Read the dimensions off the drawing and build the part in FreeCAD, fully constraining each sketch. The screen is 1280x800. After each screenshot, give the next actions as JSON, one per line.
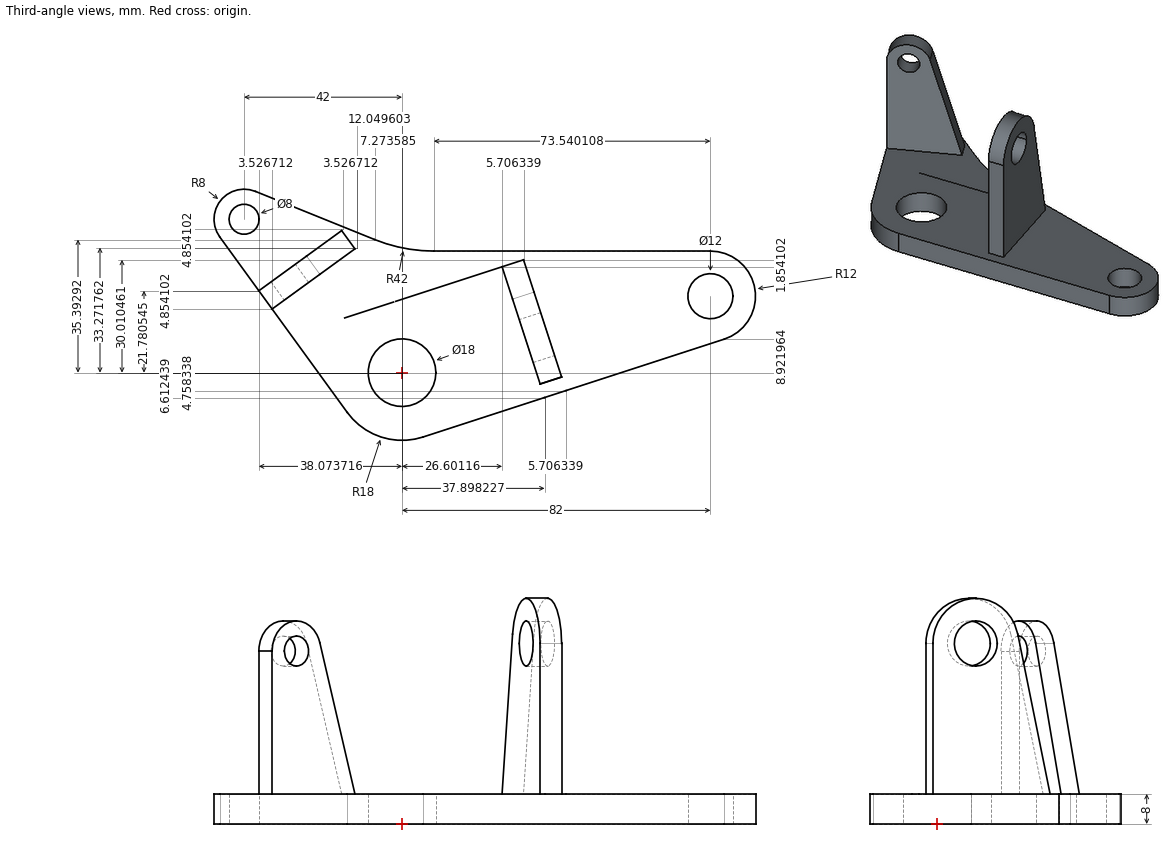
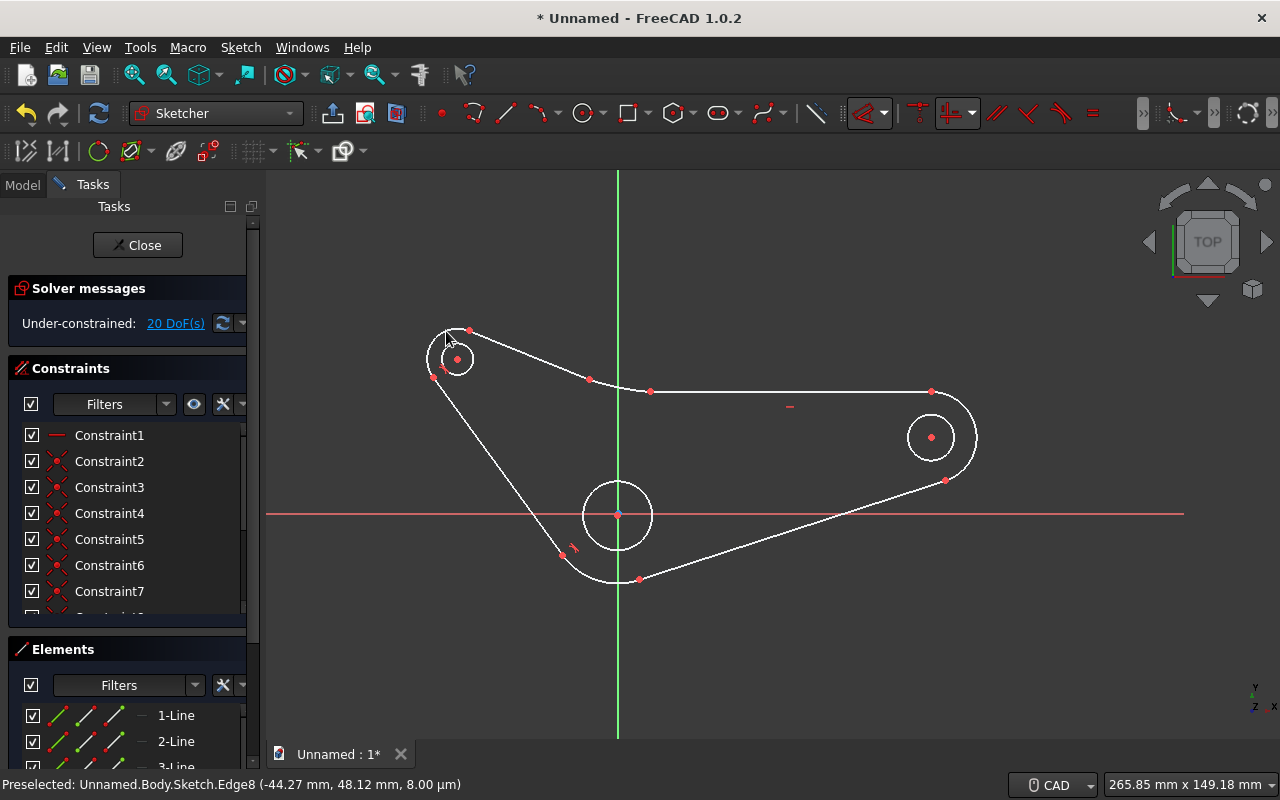
{"action": "left_click", "coordinate": [731, 550]}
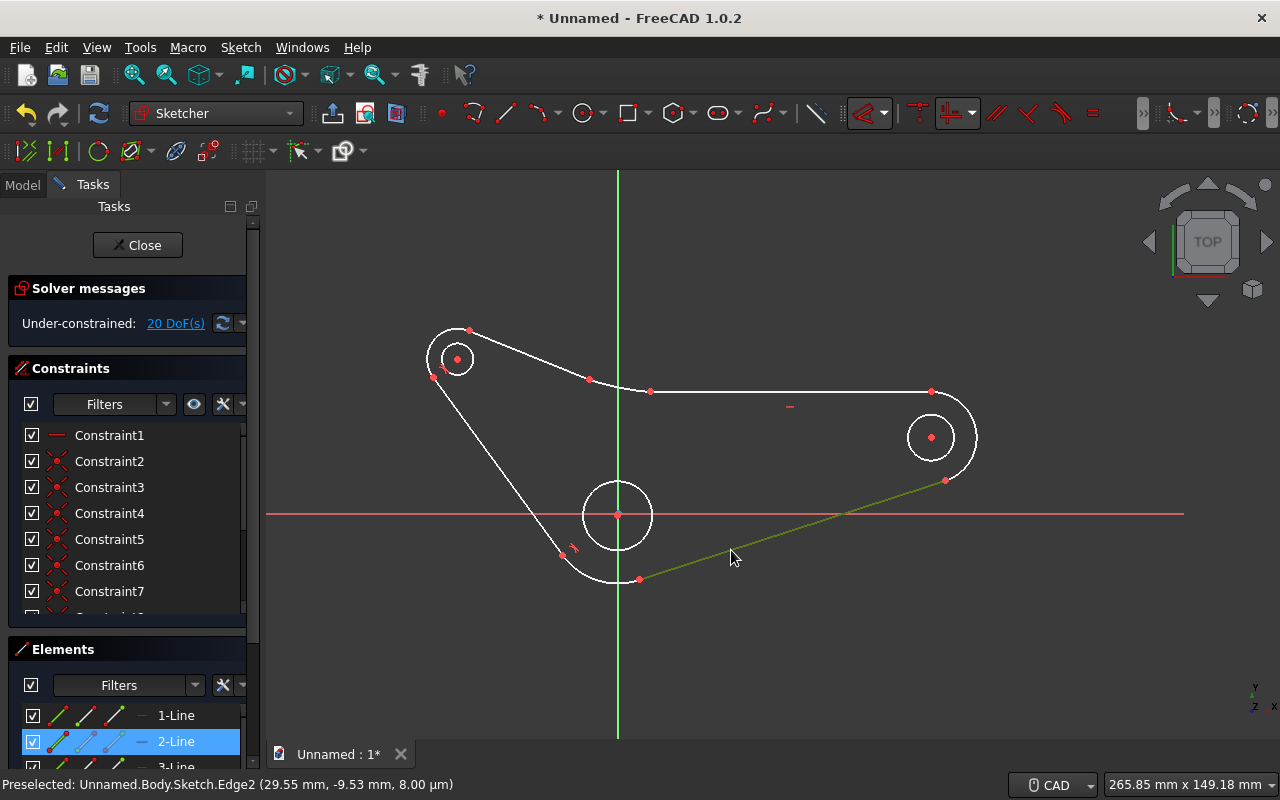
{"action": "left_click", "coordinate": [582, 573]}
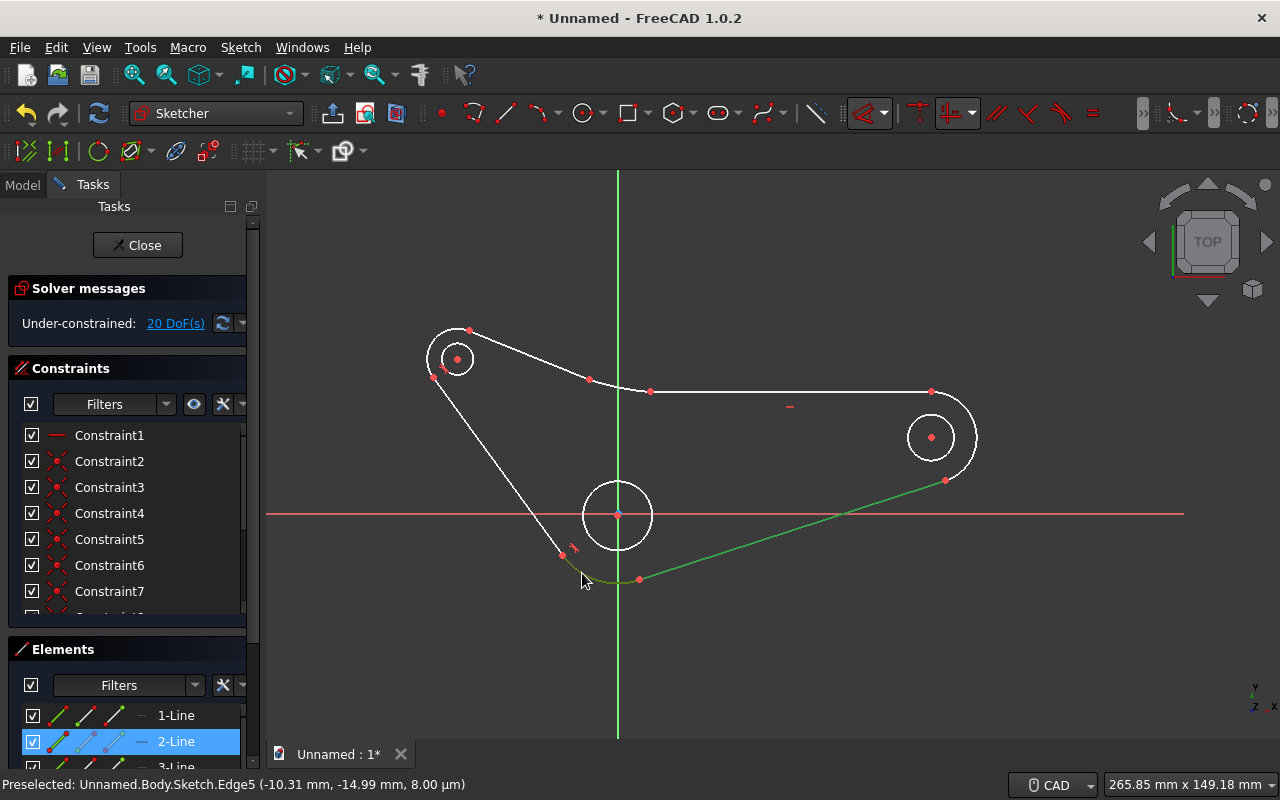
{"action": "key", "text": "t"}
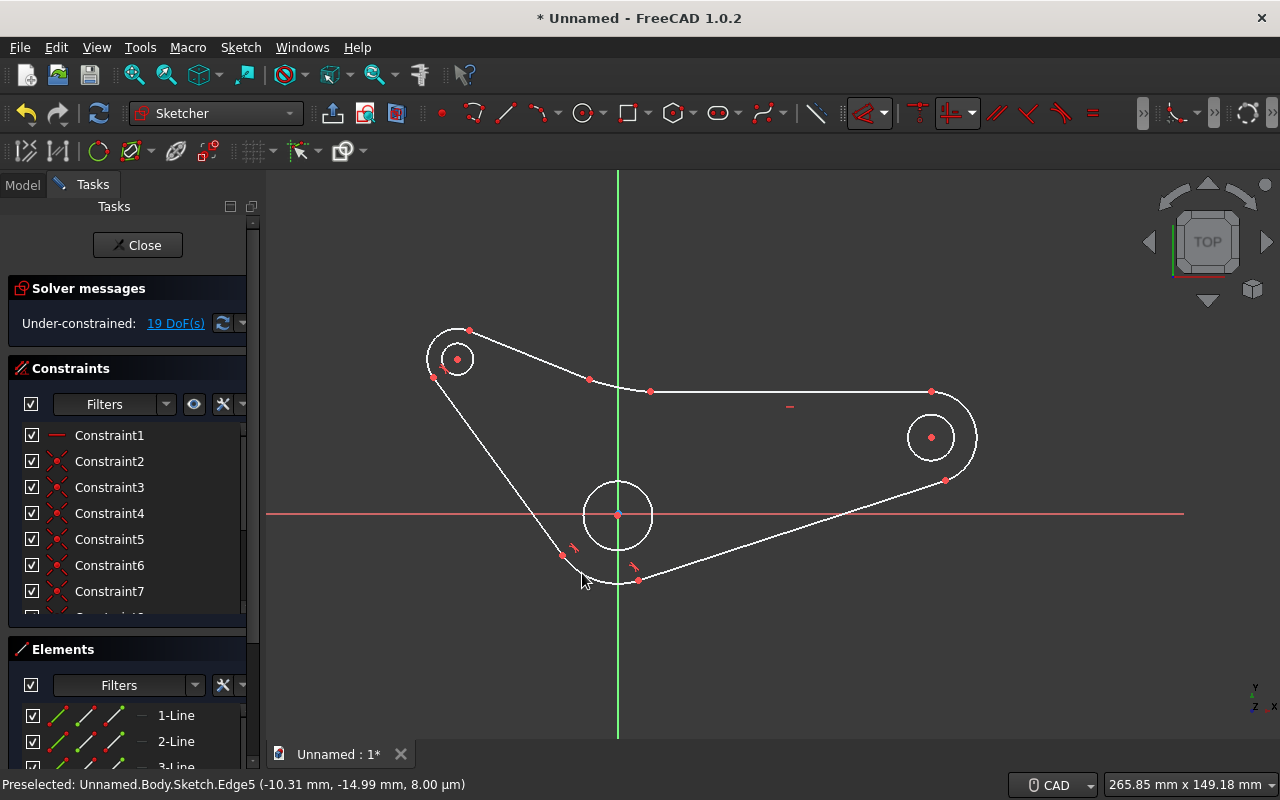
{"action": "left_click", "coordinate": [731, 551]}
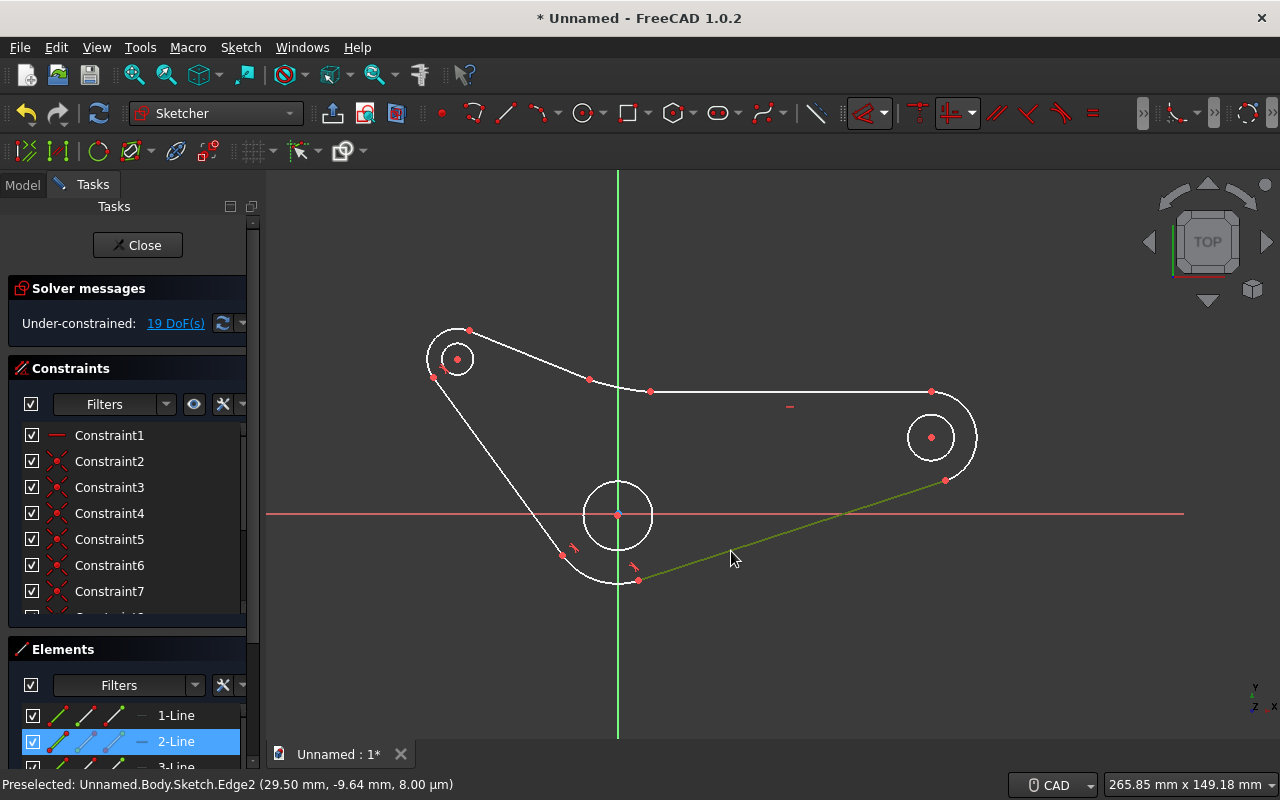
{"action": "left_click", "coordinate": [973, 456]}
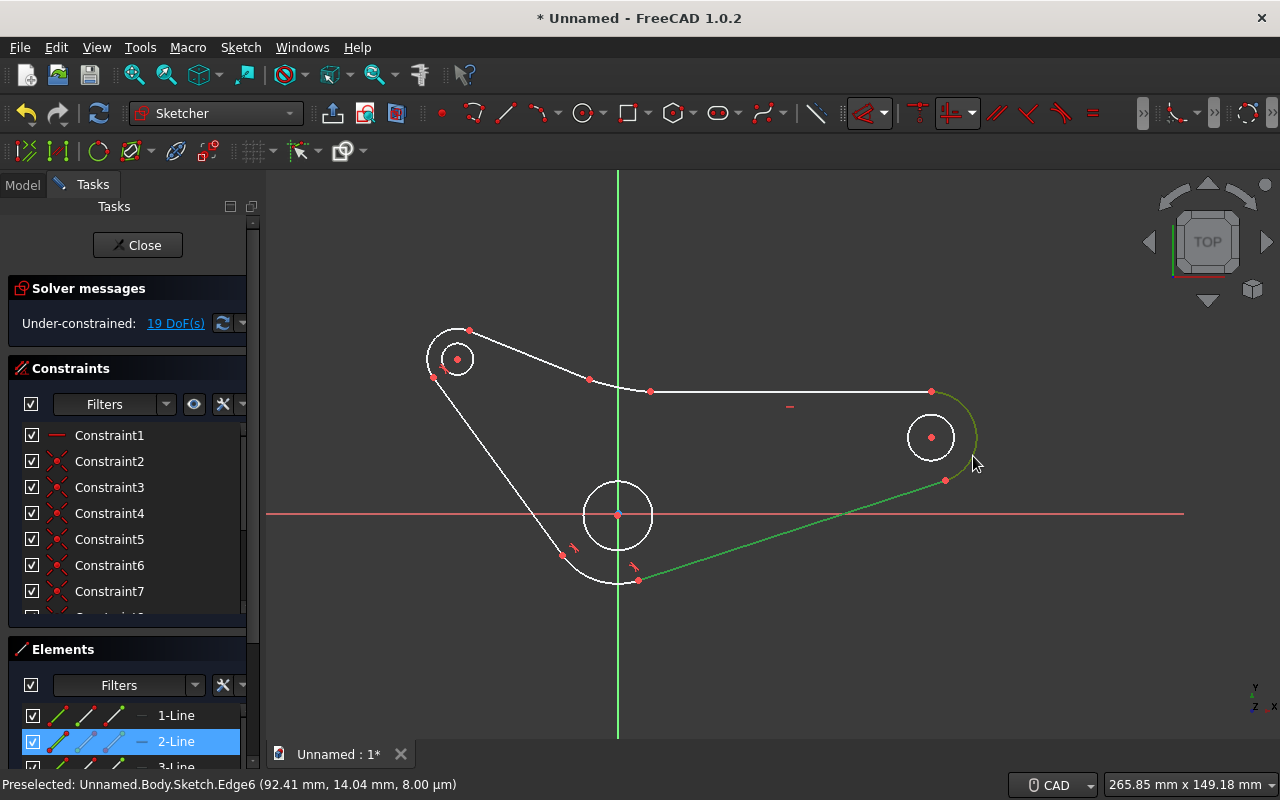
{"action": "key", "text": "t"}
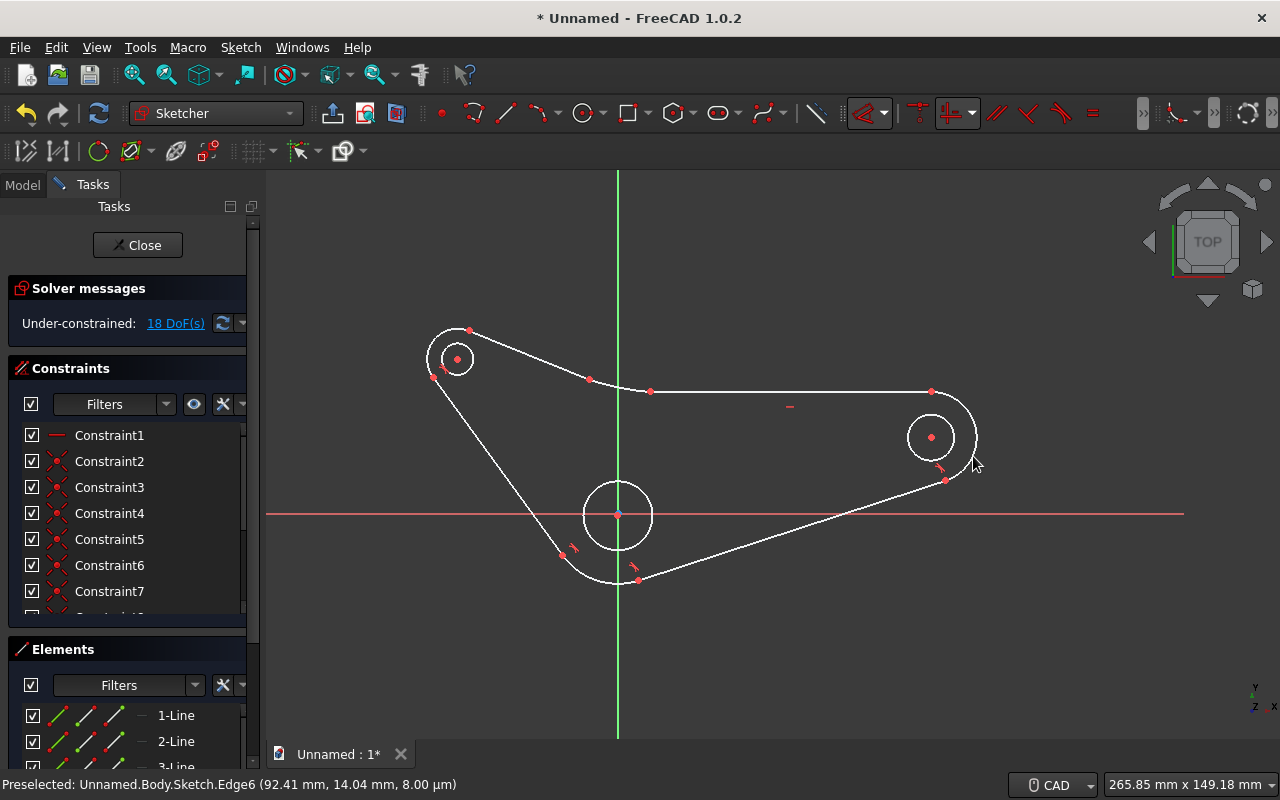
{"action": "left_click", "coordinate": [847, 392]}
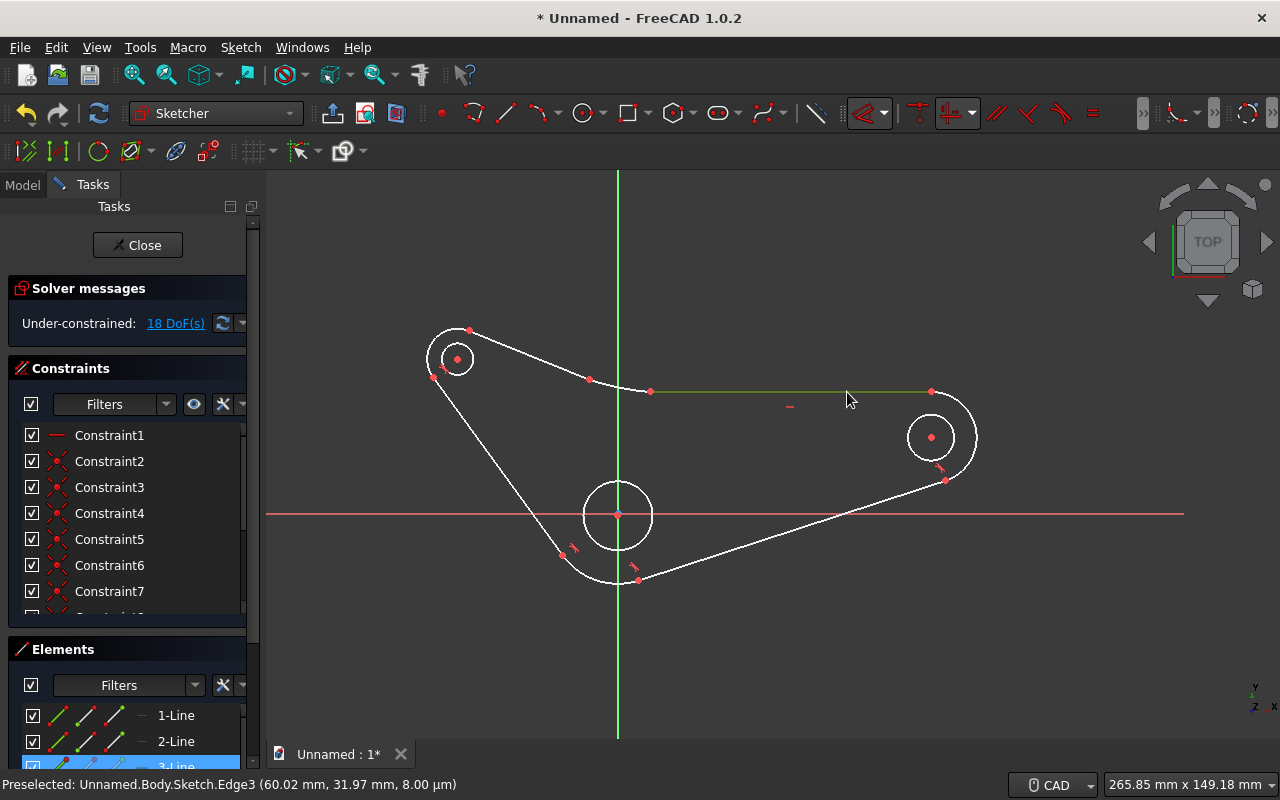
{"action": "left_click", "coordinate": [973, 456]}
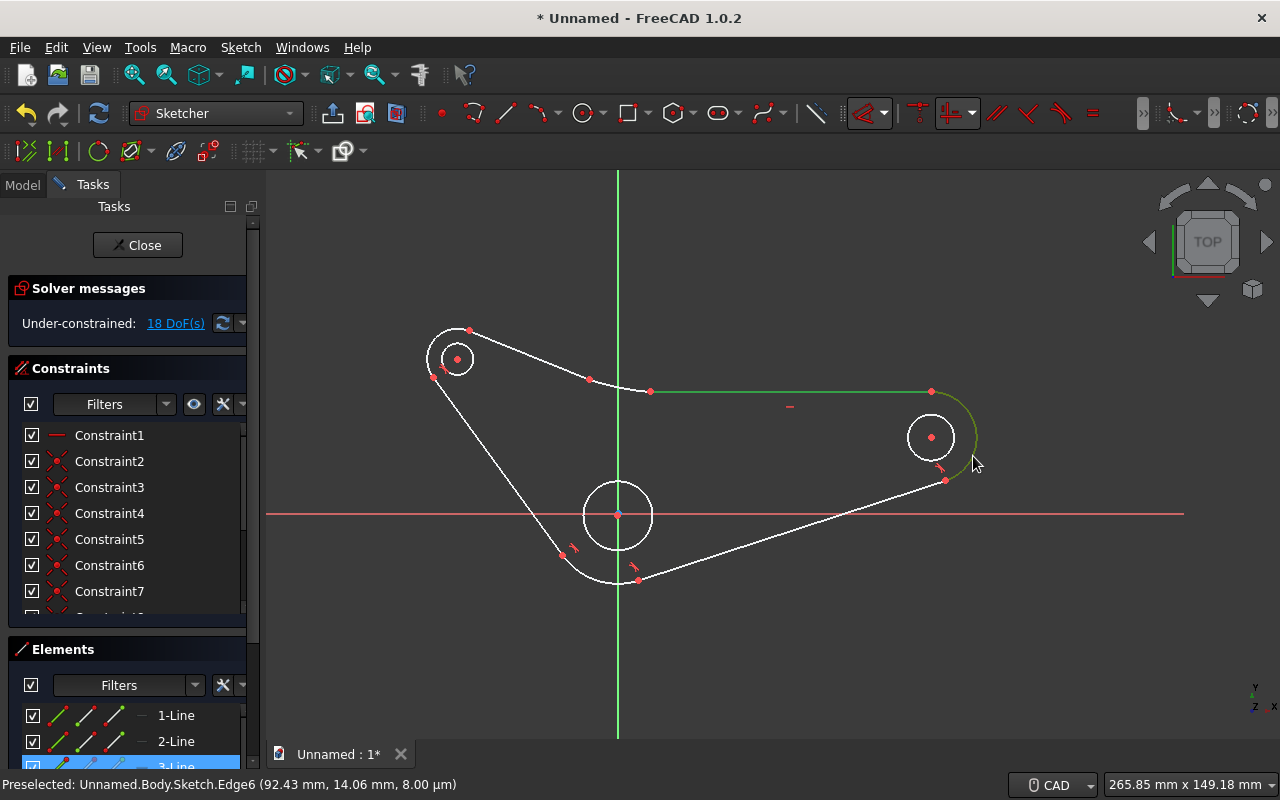
{"action": "left_click", "coordinate": [1062, 114]}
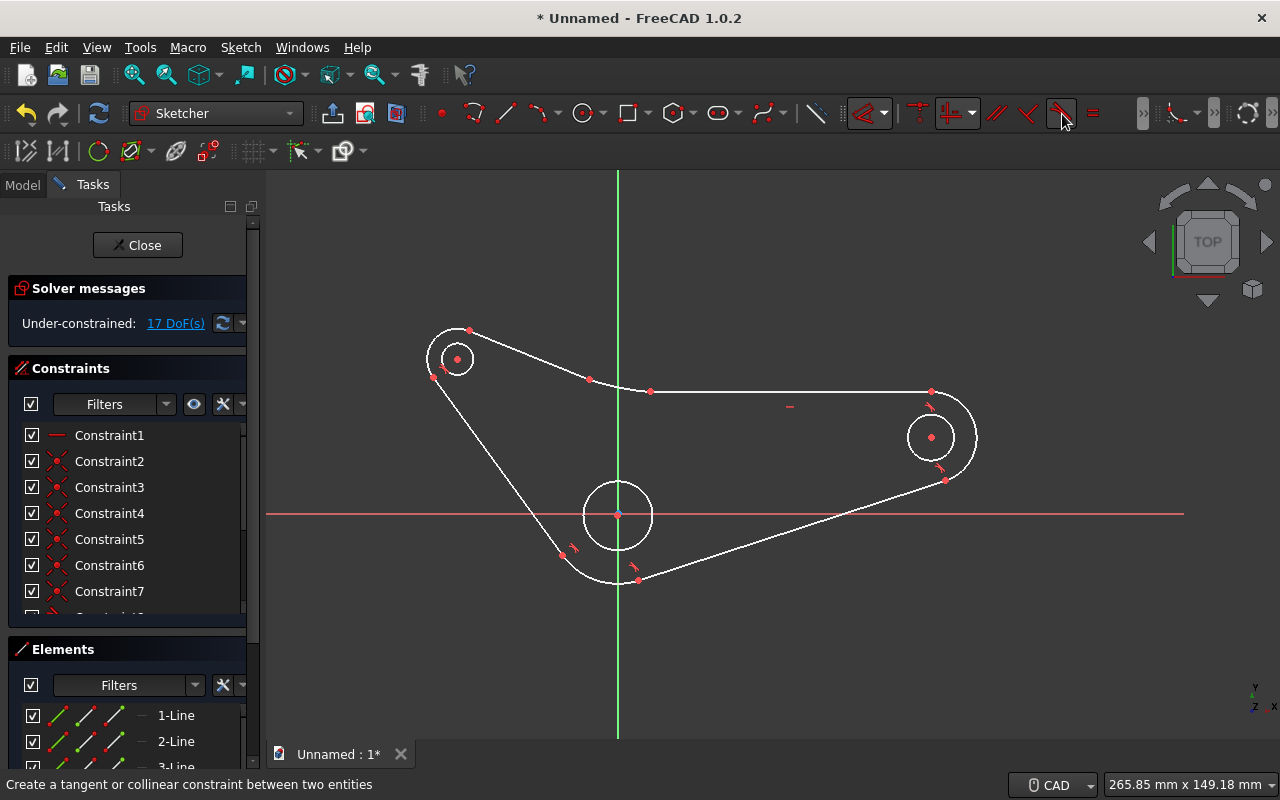
{"action": "left_click", "coordinate": [554, 365]}